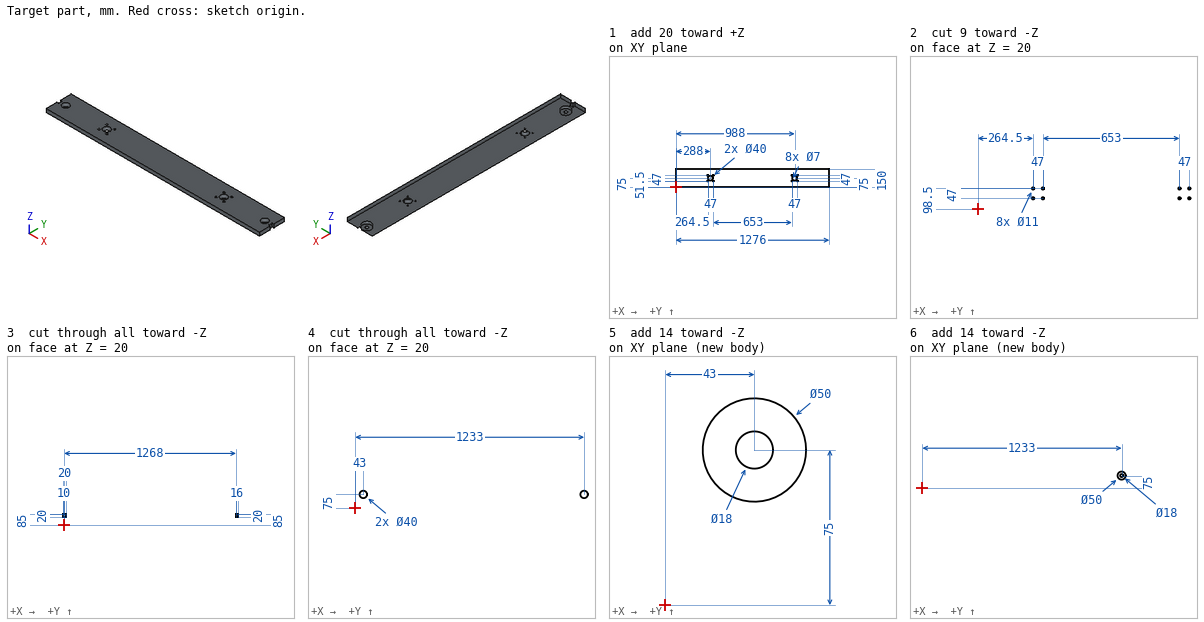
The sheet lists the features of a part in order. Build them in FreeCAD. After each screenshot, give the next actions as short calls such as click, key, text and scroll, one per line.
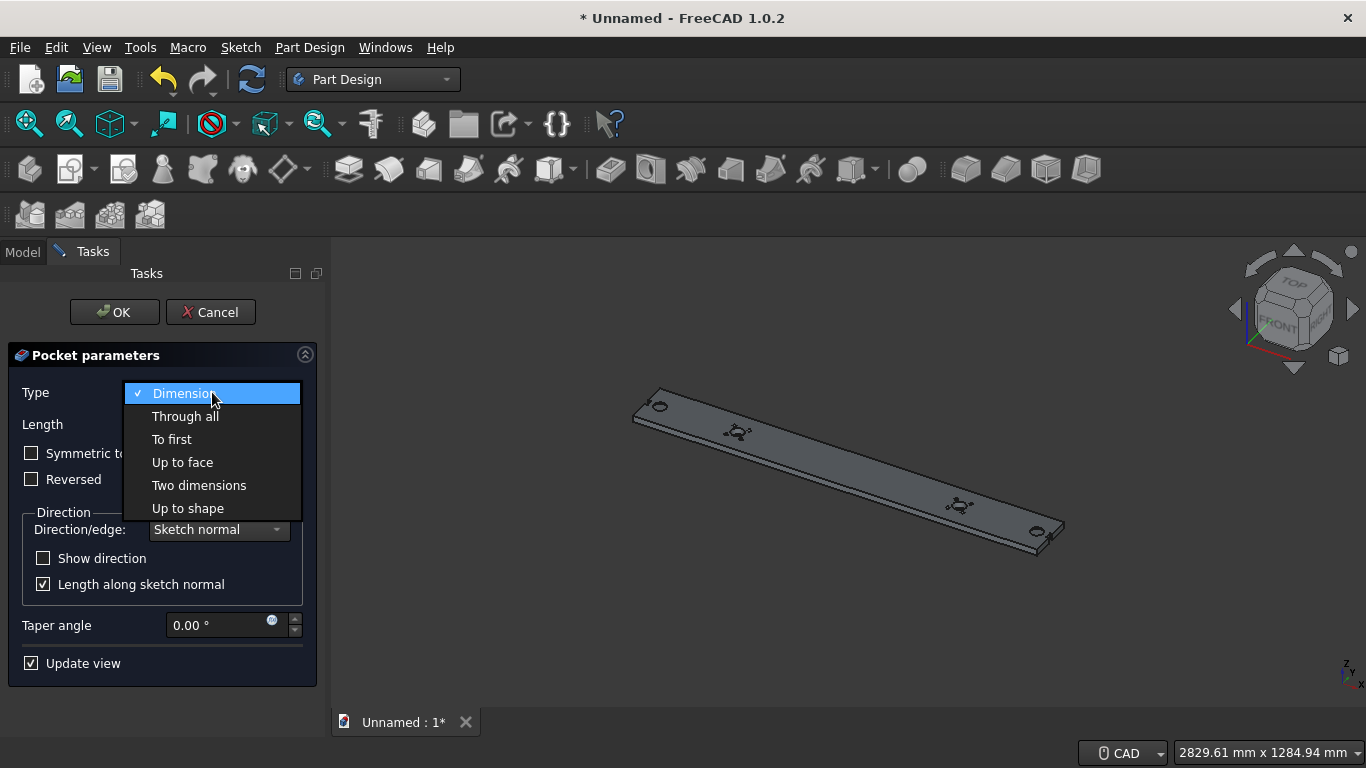
click(212, 416)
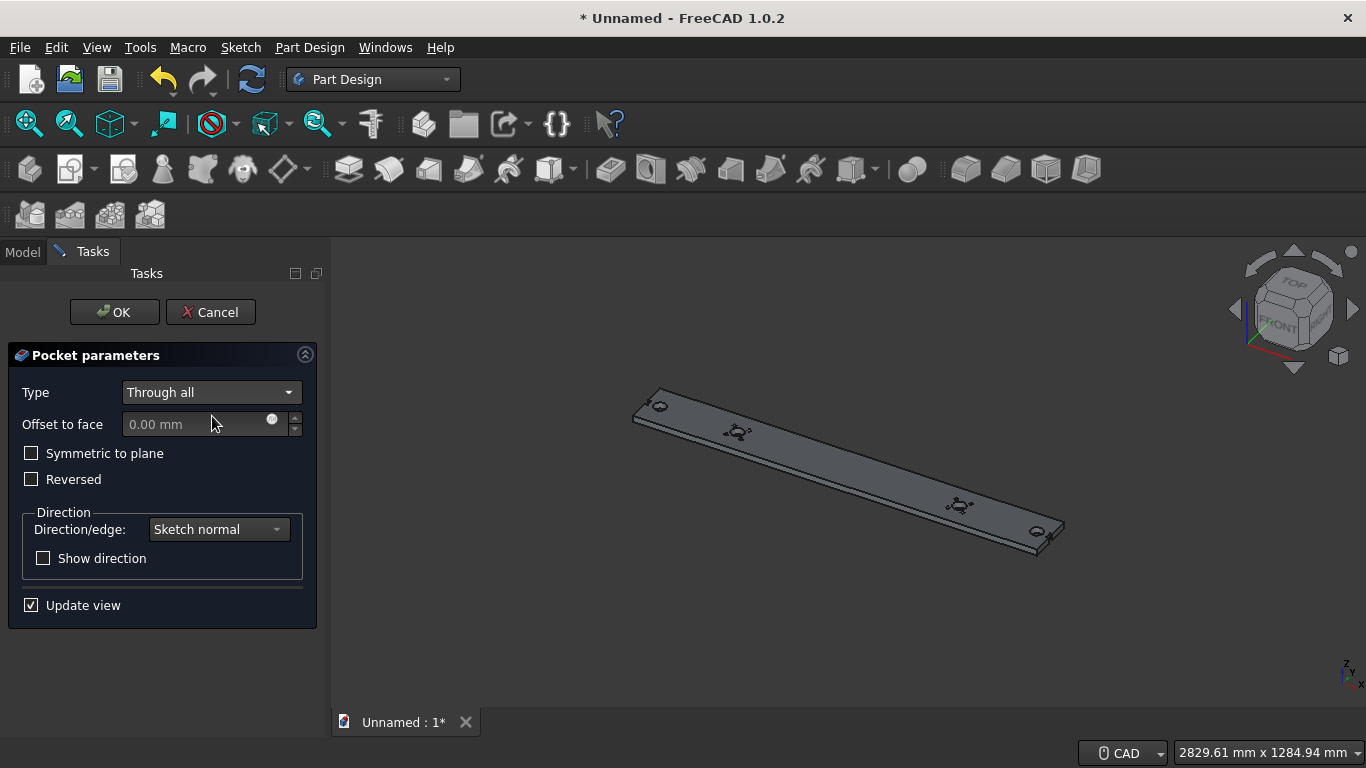
click(115, 312)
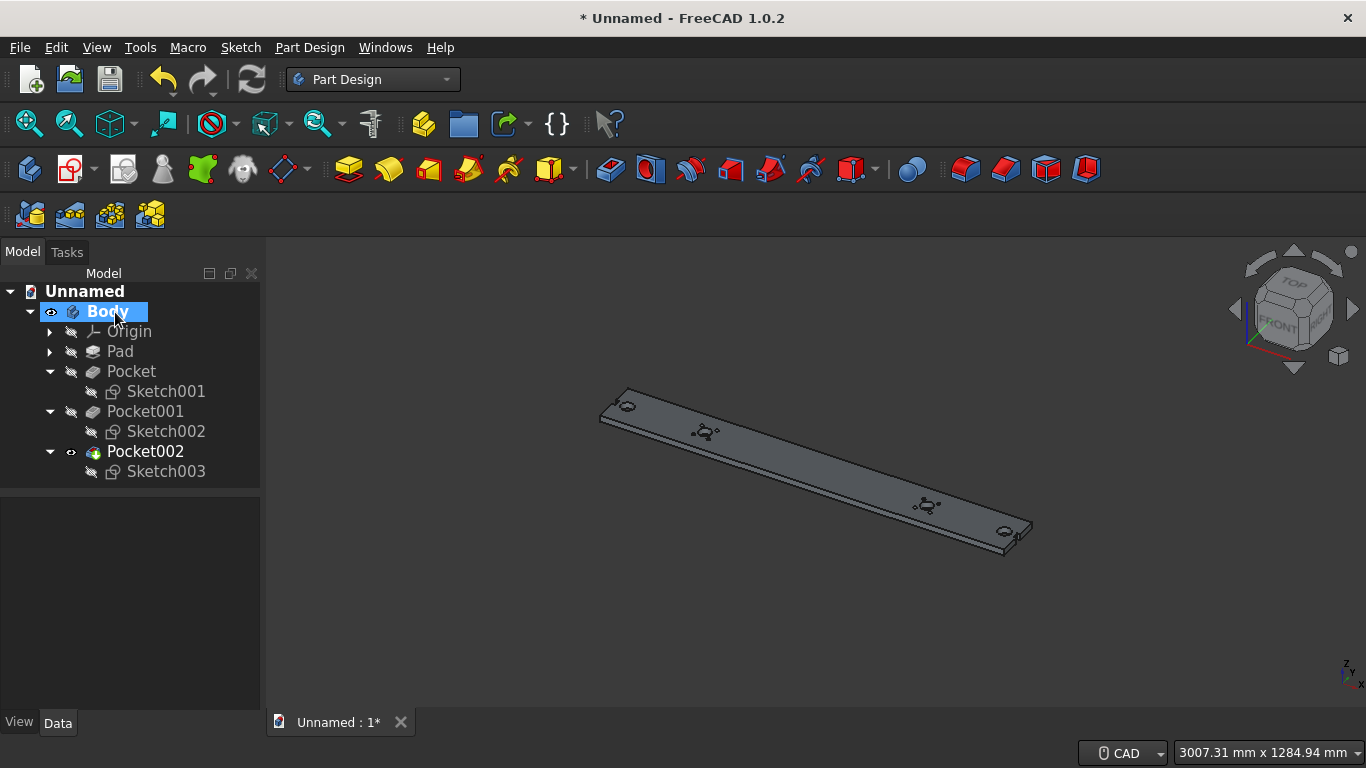
click(30, 124)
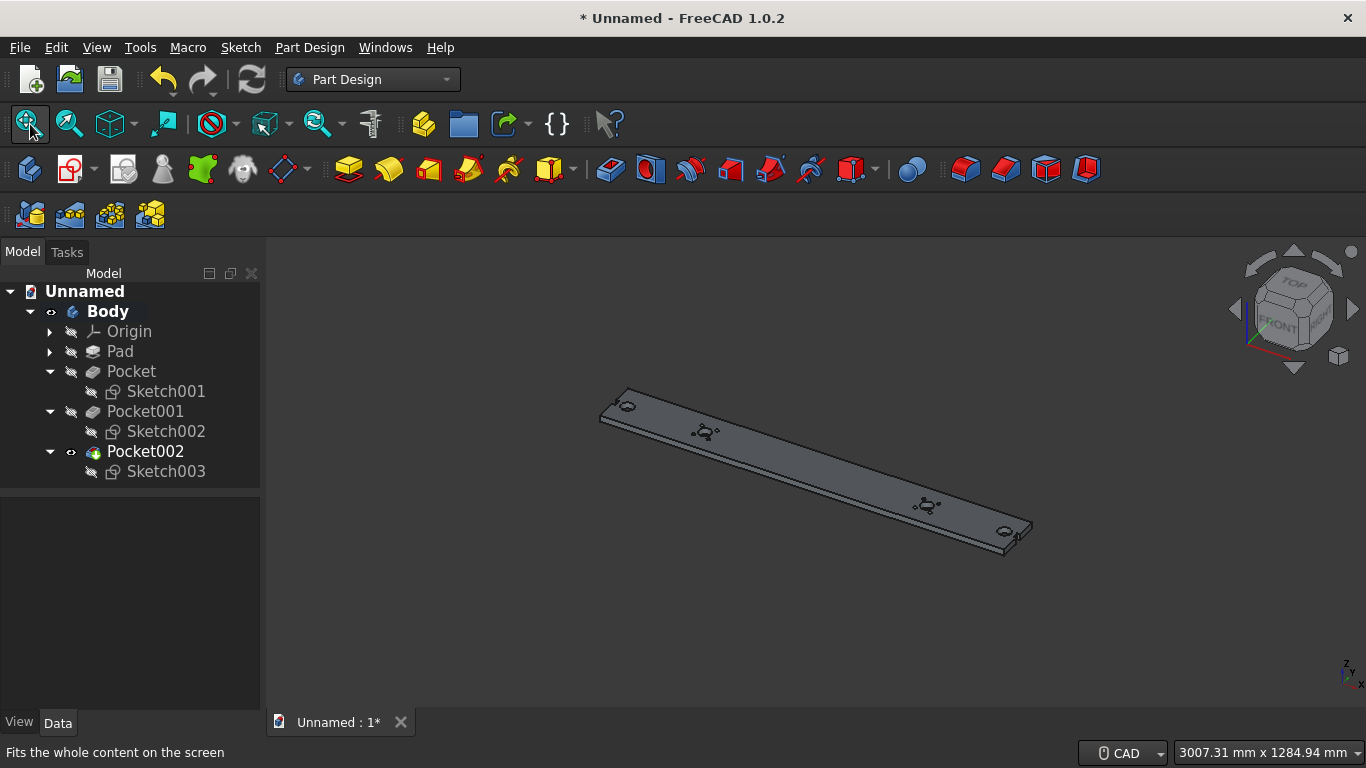
click(30, 170)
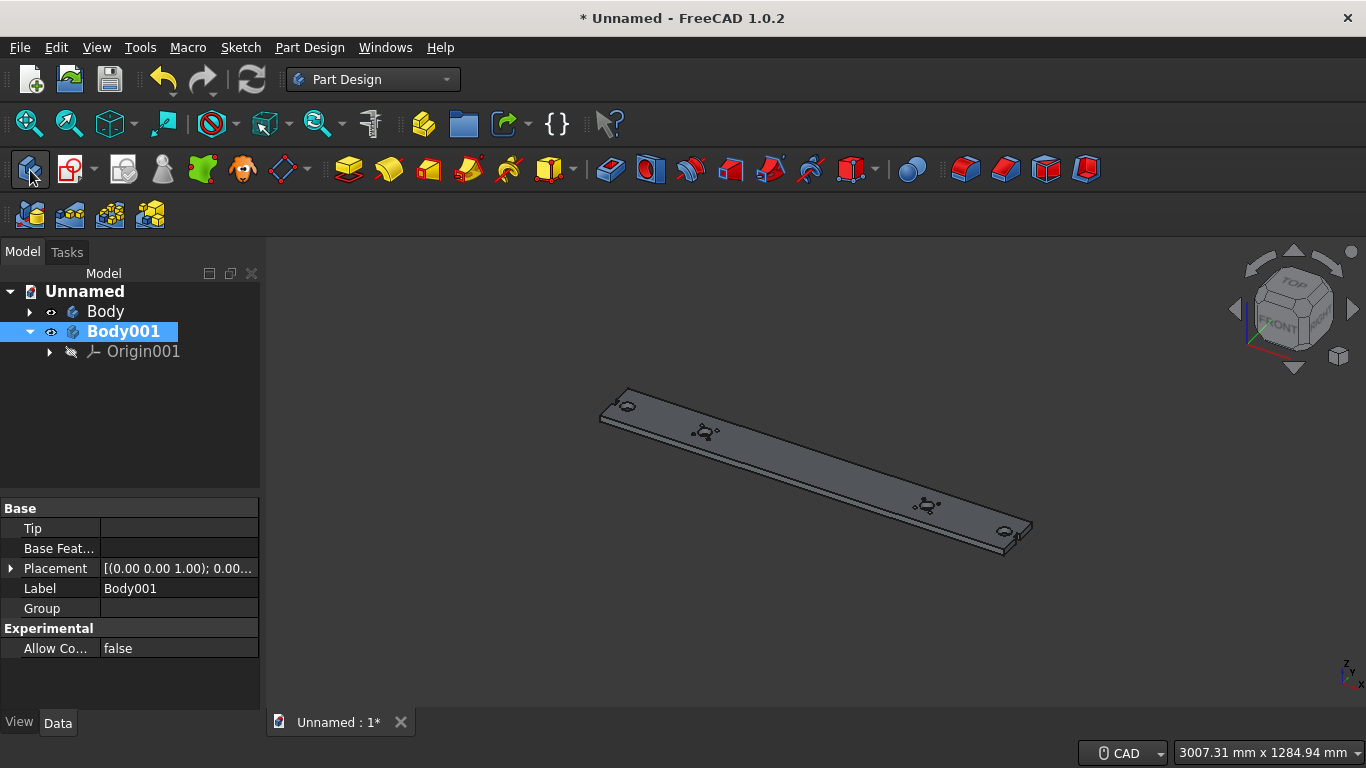
click(306, 667)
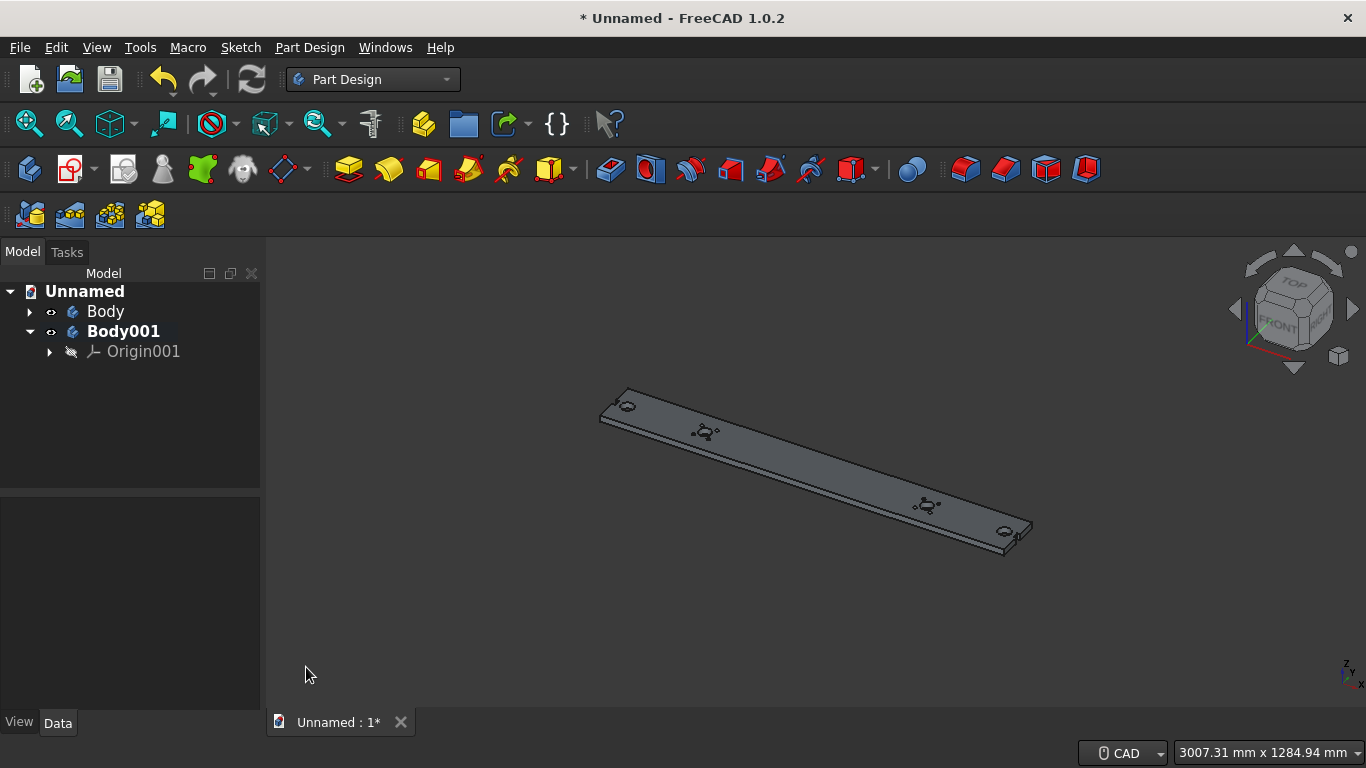
click(70, 170)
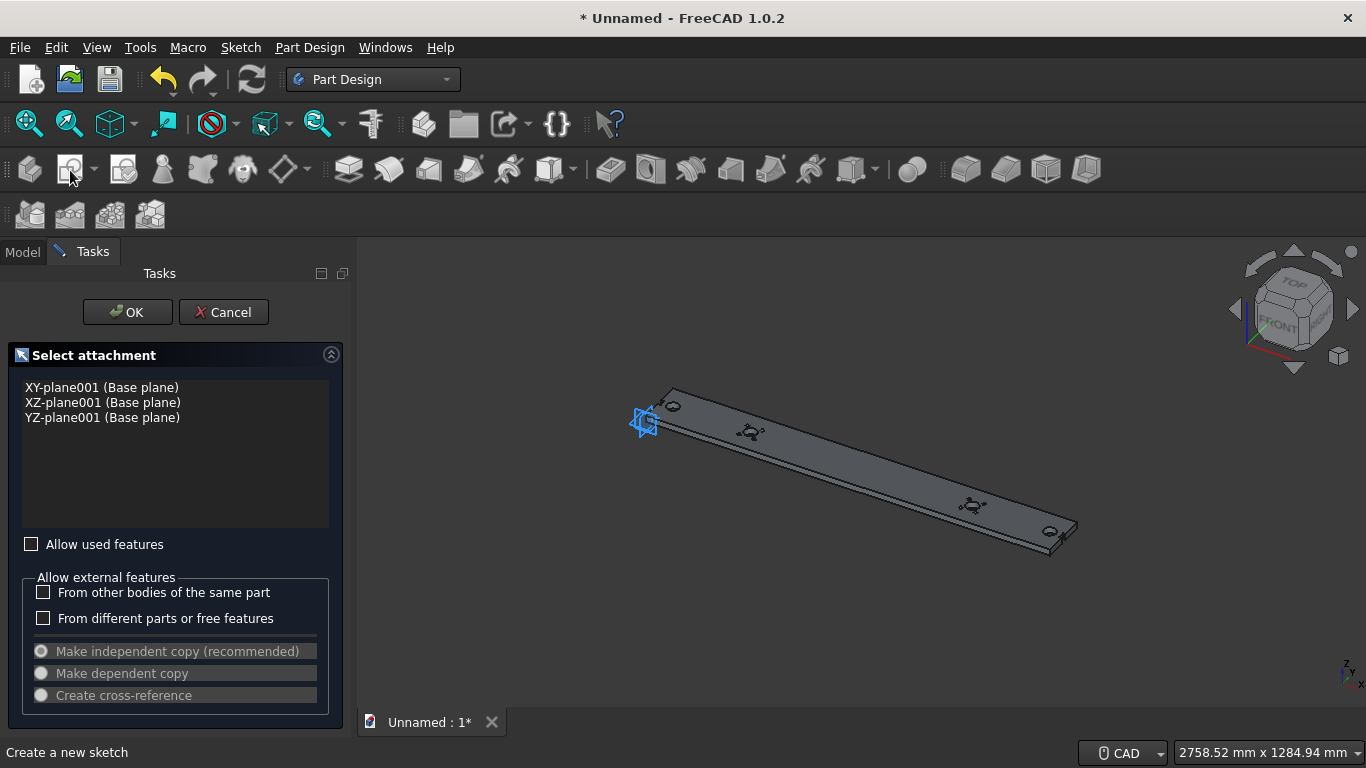
click(82, 388)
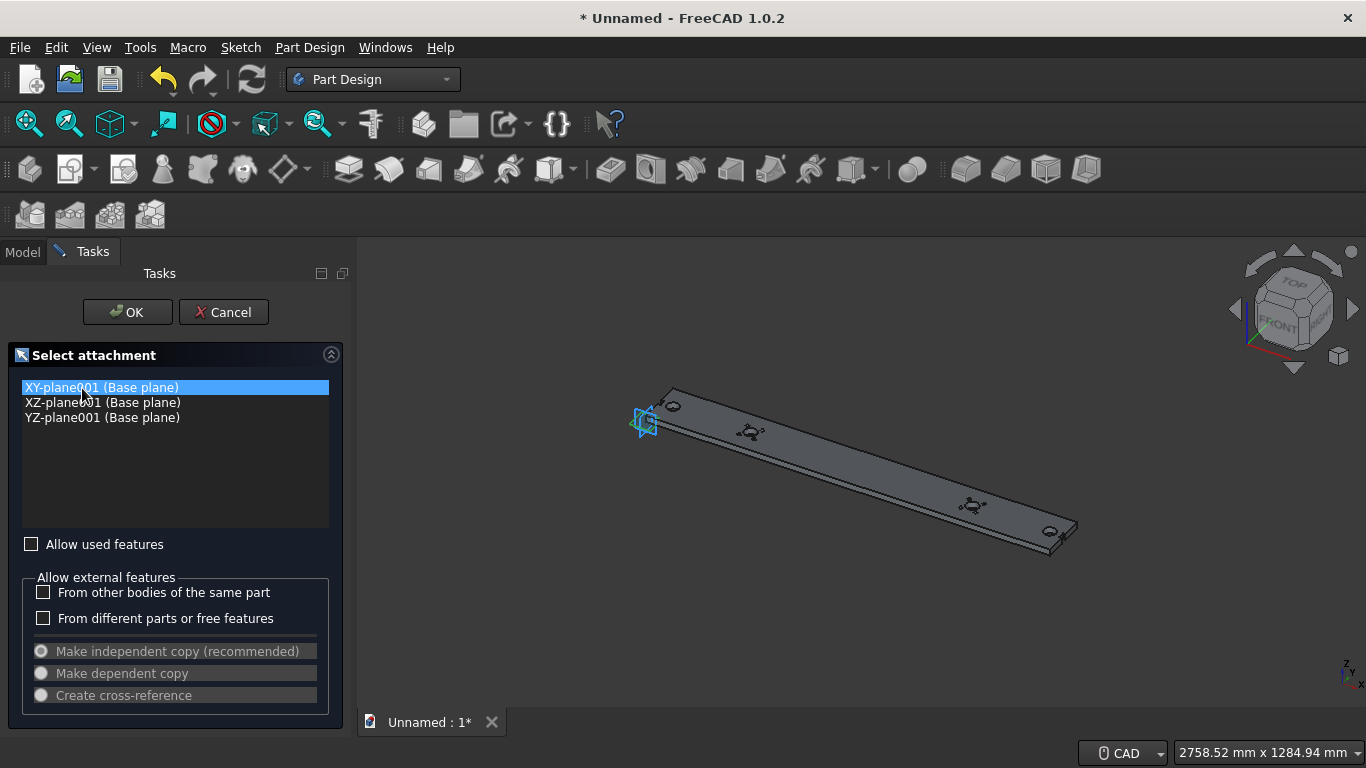
click(128, 312)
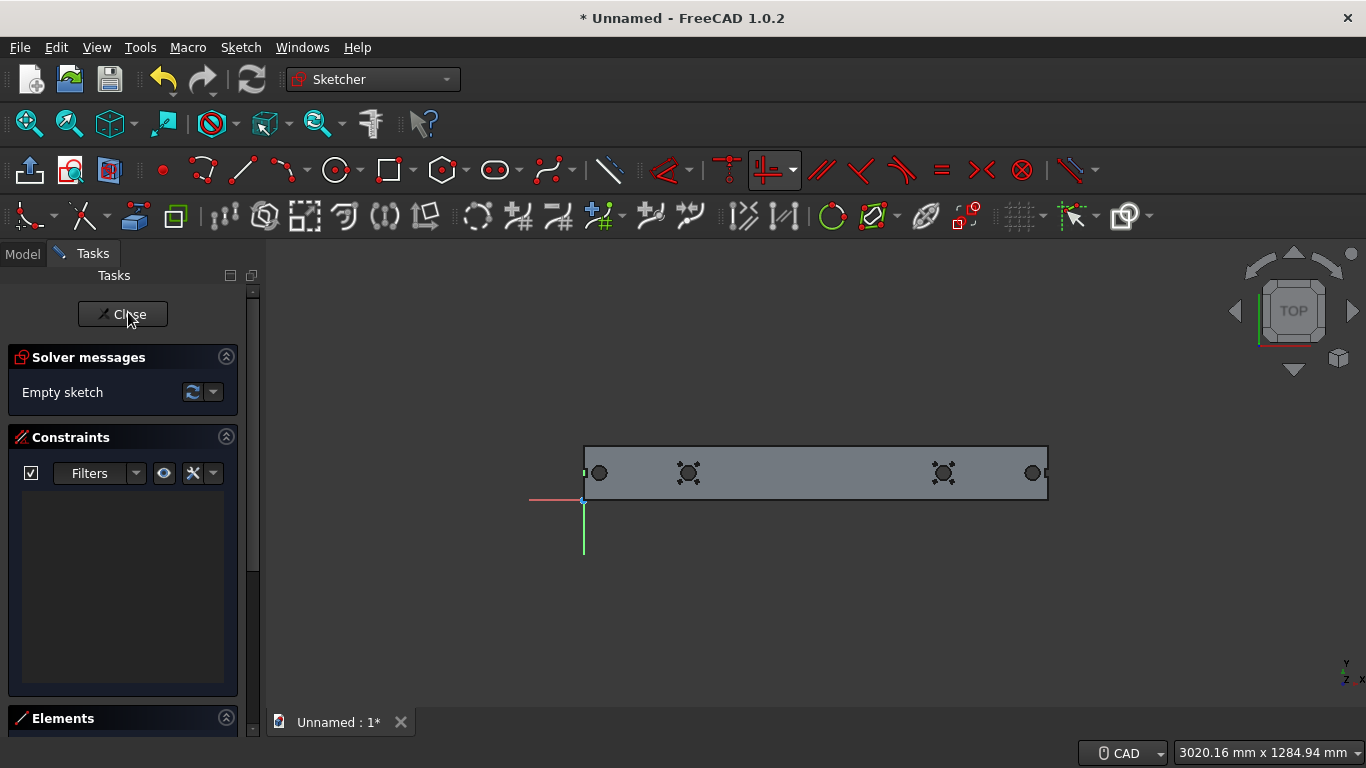
scroll(572, 484, up, 10)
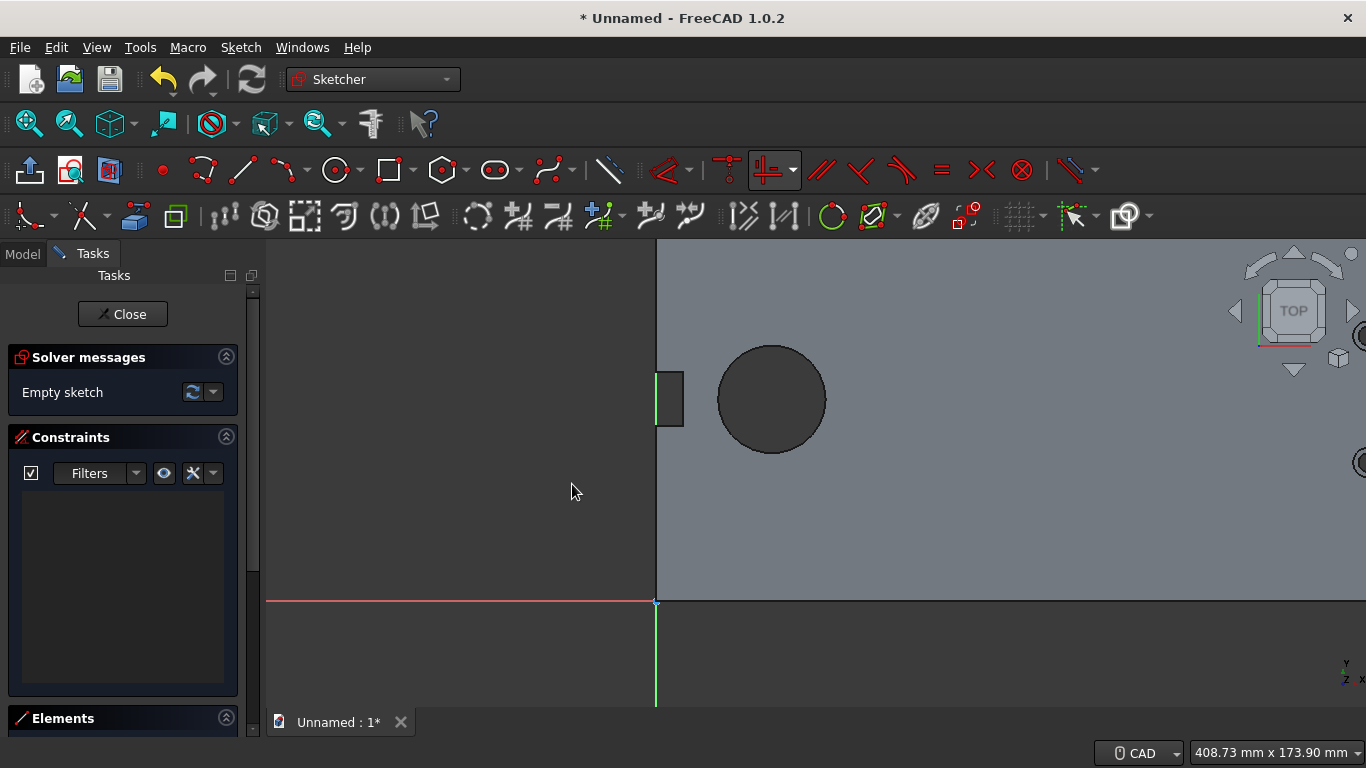
click(336, 170)